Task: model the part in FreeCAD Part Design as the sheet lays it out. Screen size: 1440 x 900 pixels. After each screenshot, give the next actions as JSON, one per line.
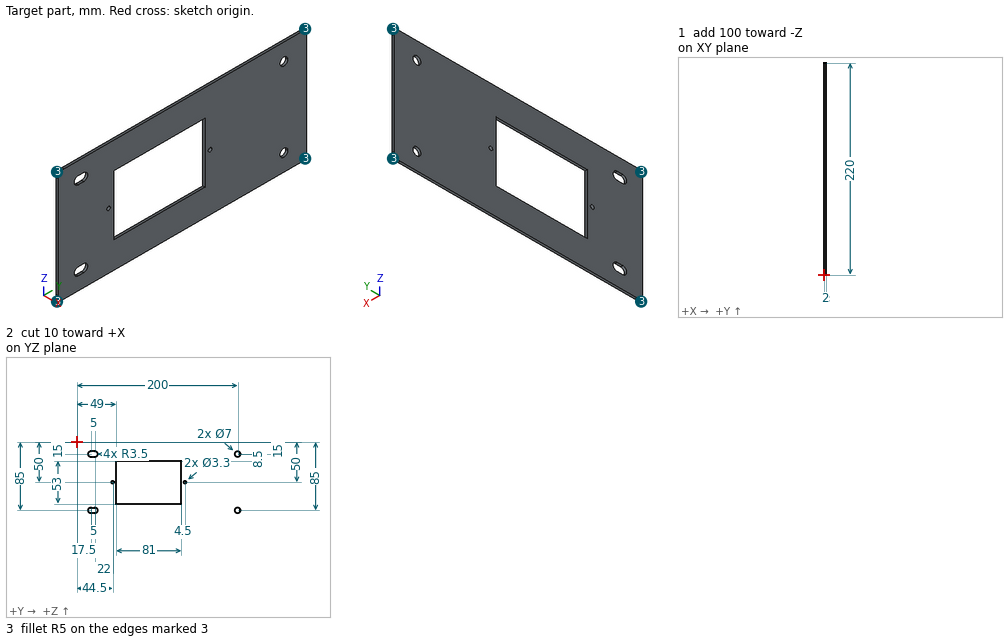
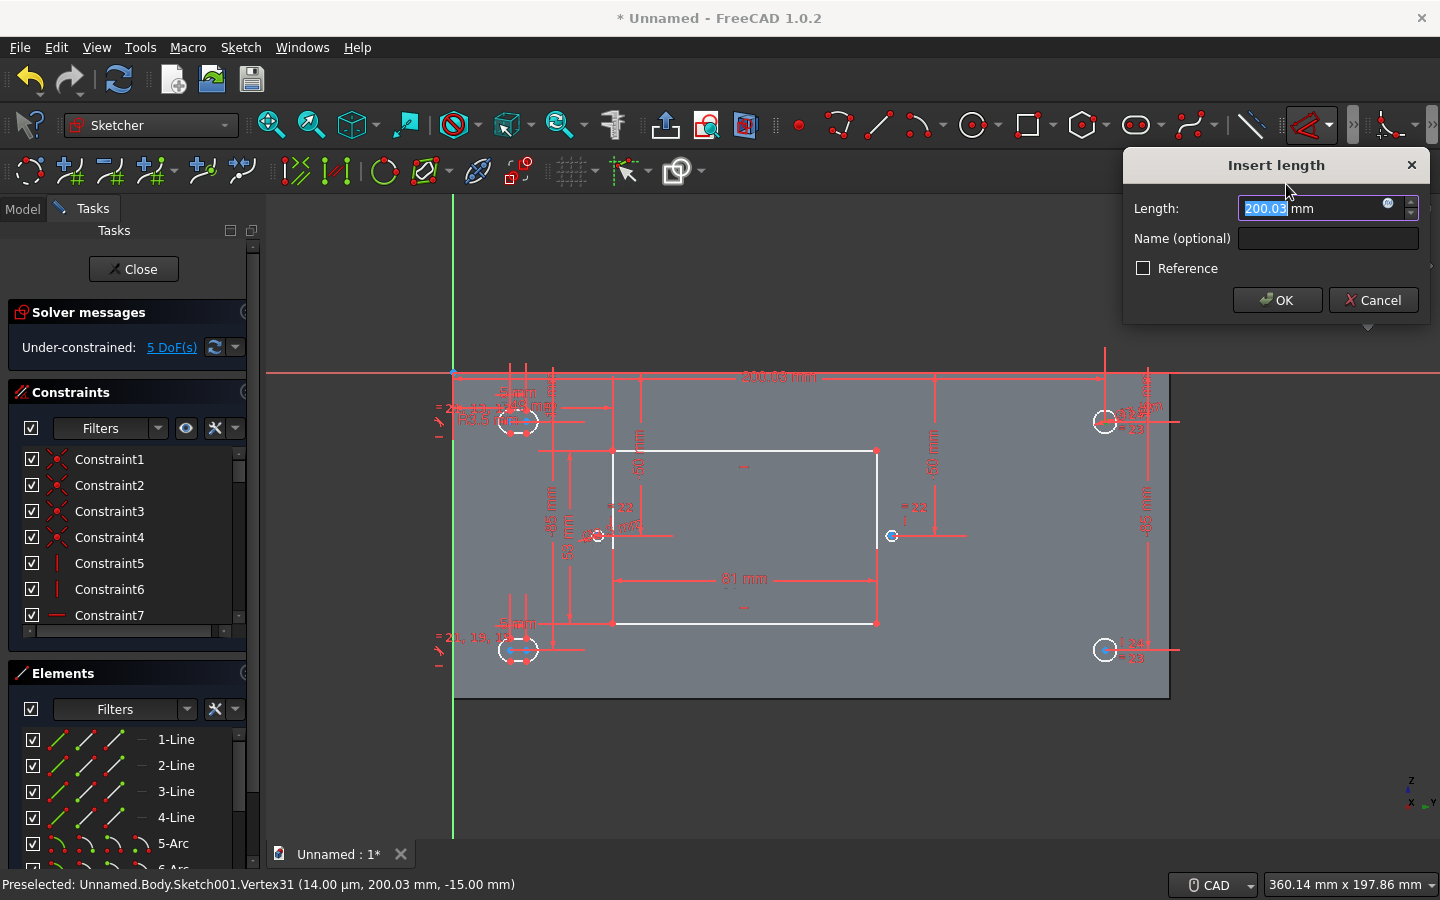
{"action": "type", "text": "200"}
{"action": "key", "text": "Return"}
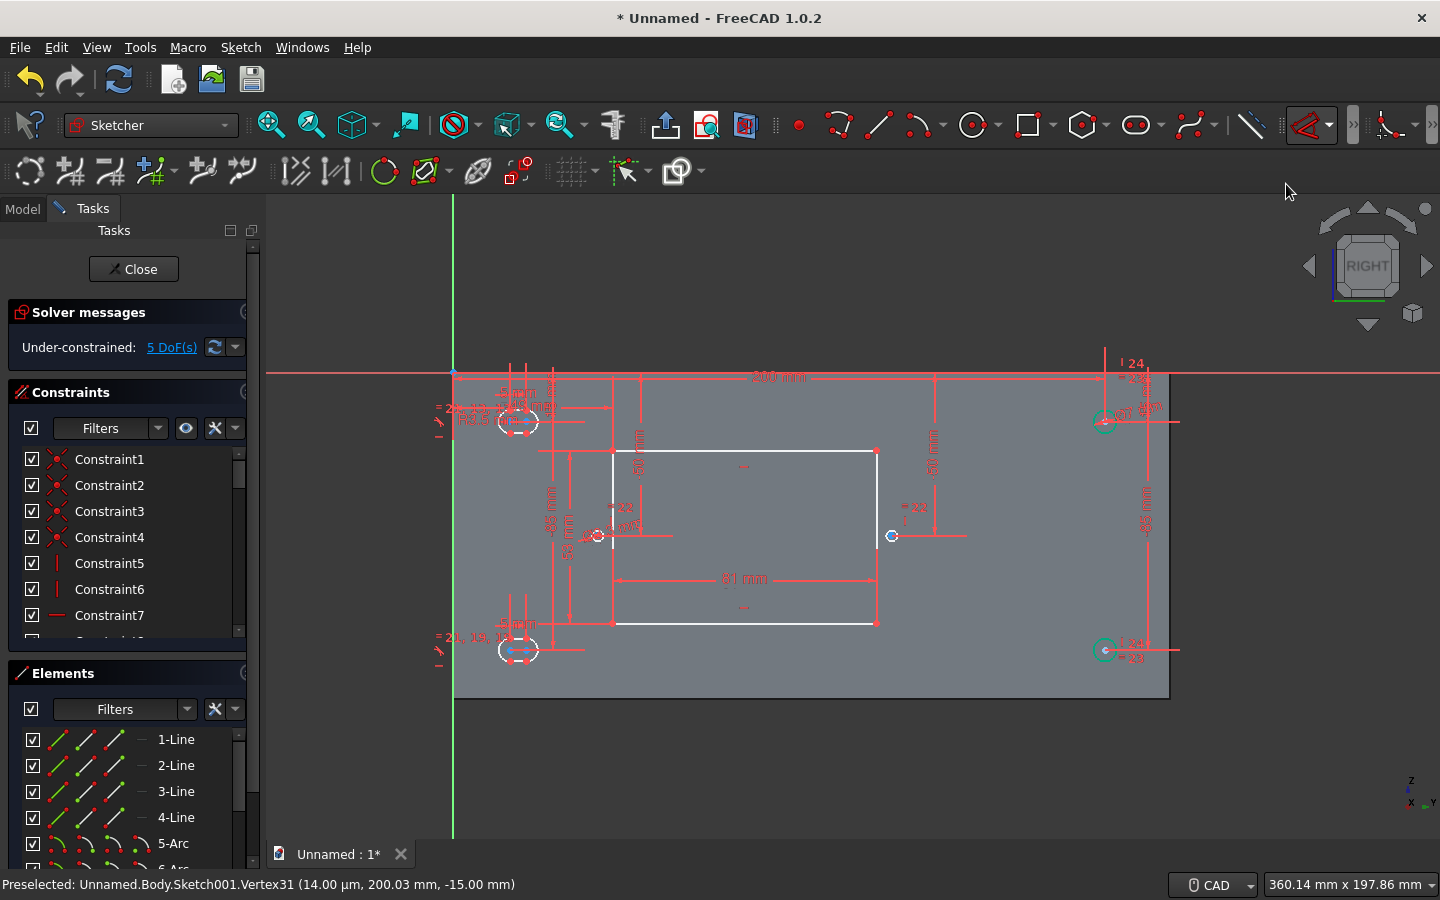
{"action": "left_click", "coordinate": [526, 433]}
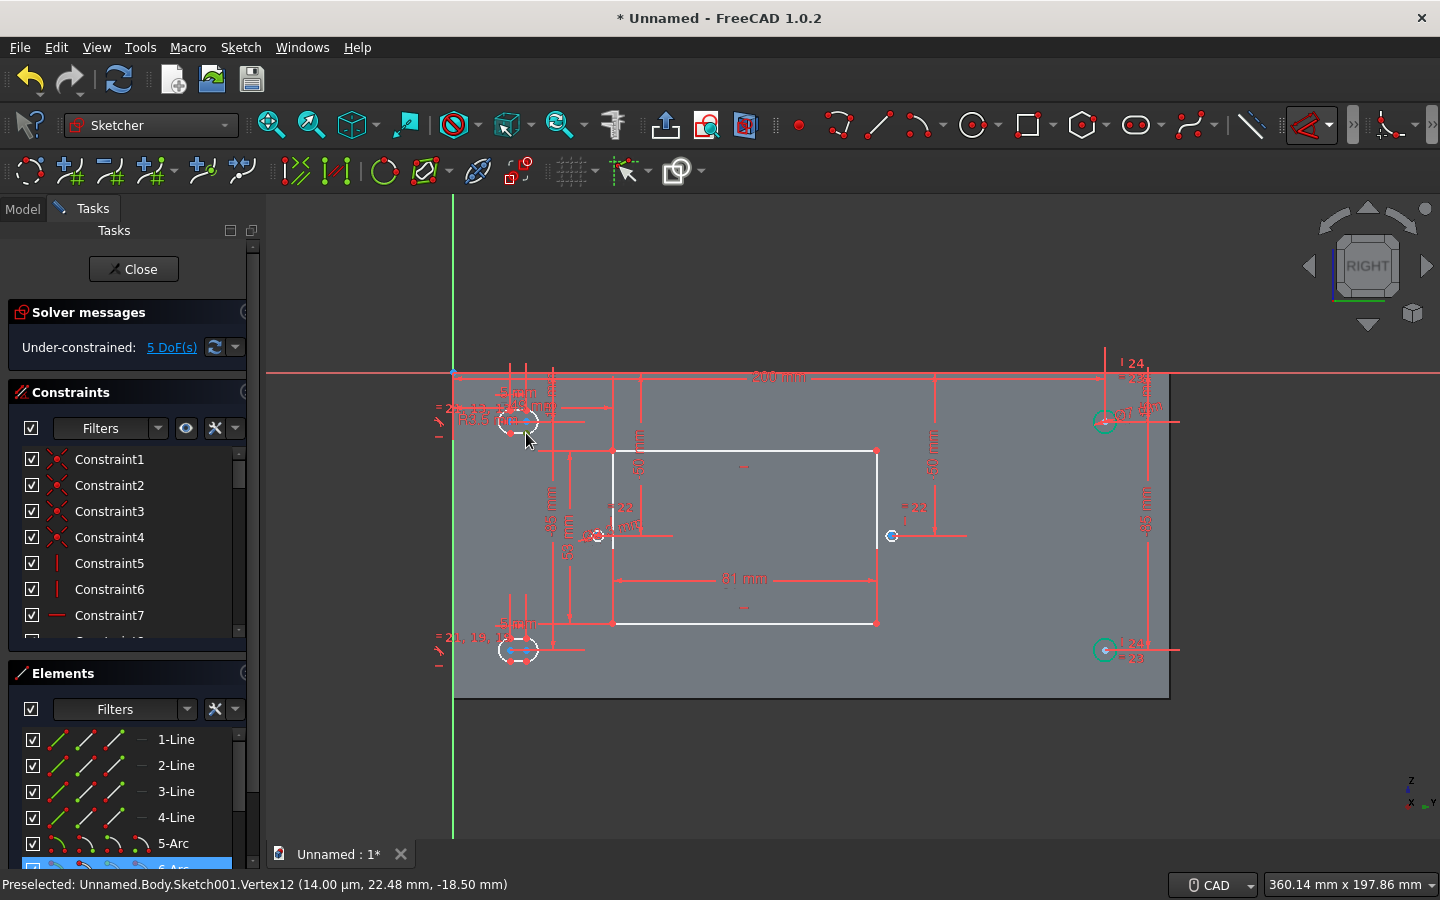
{"action": "left_click", "coordinate": [598, 536]}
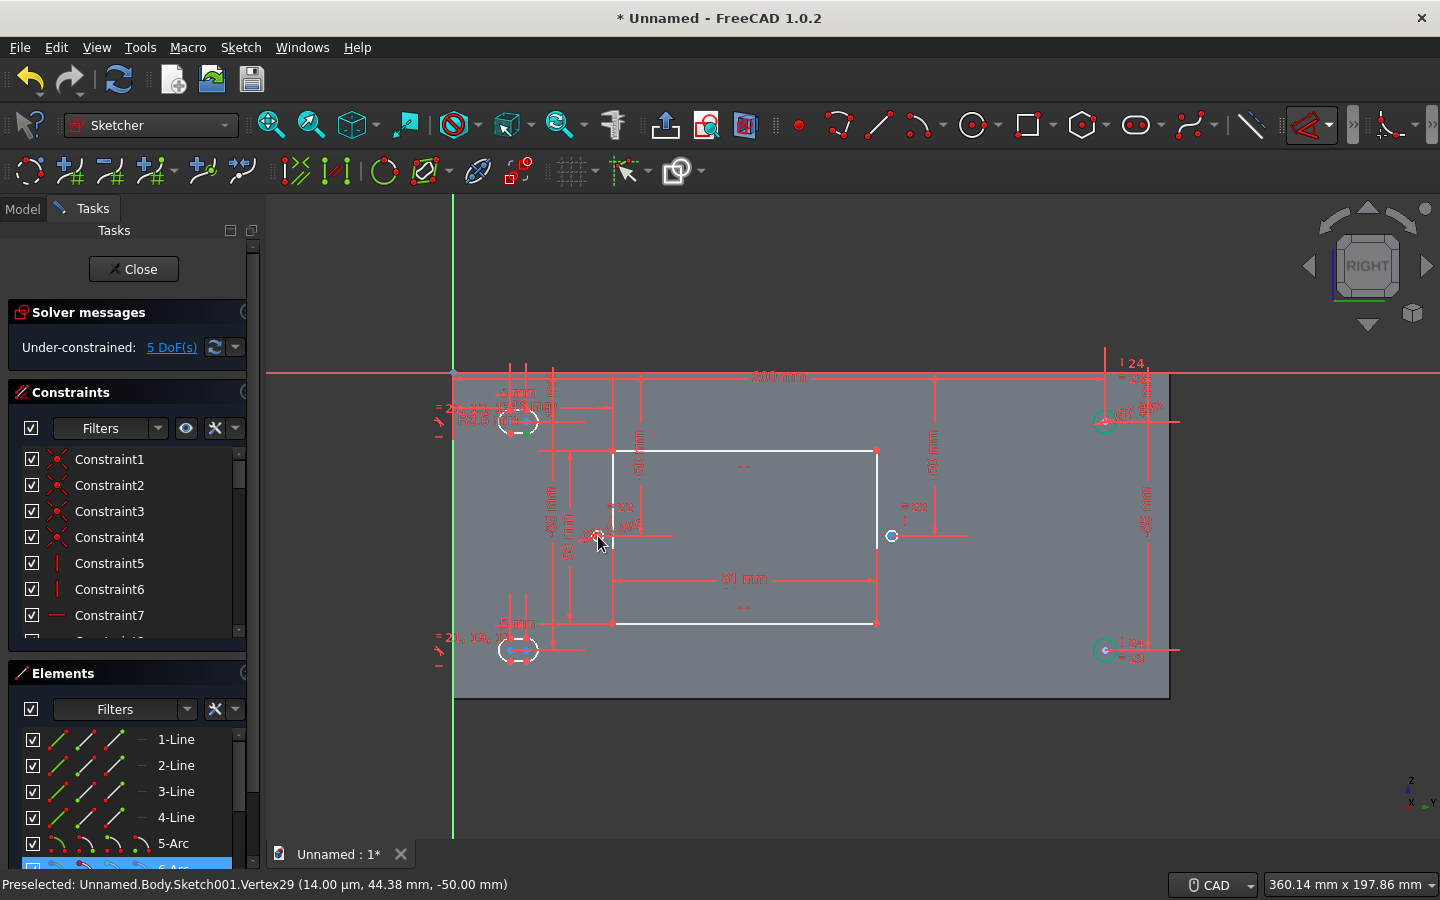
{"action": "left_click", "coordinate": [1332, 126]}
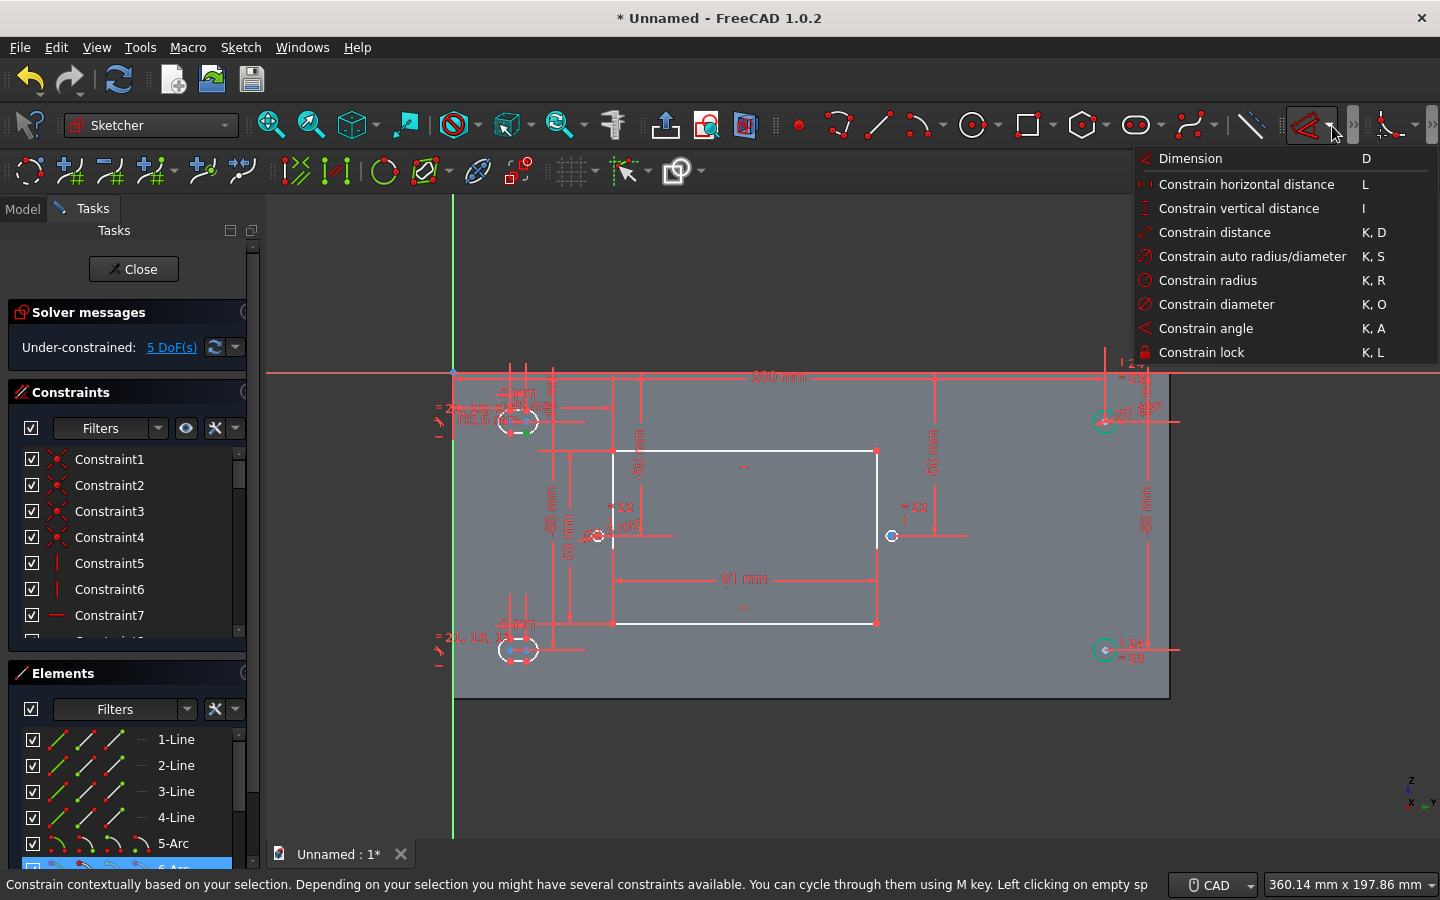
{"action": "left_click", "coordinate": [1286, 184]}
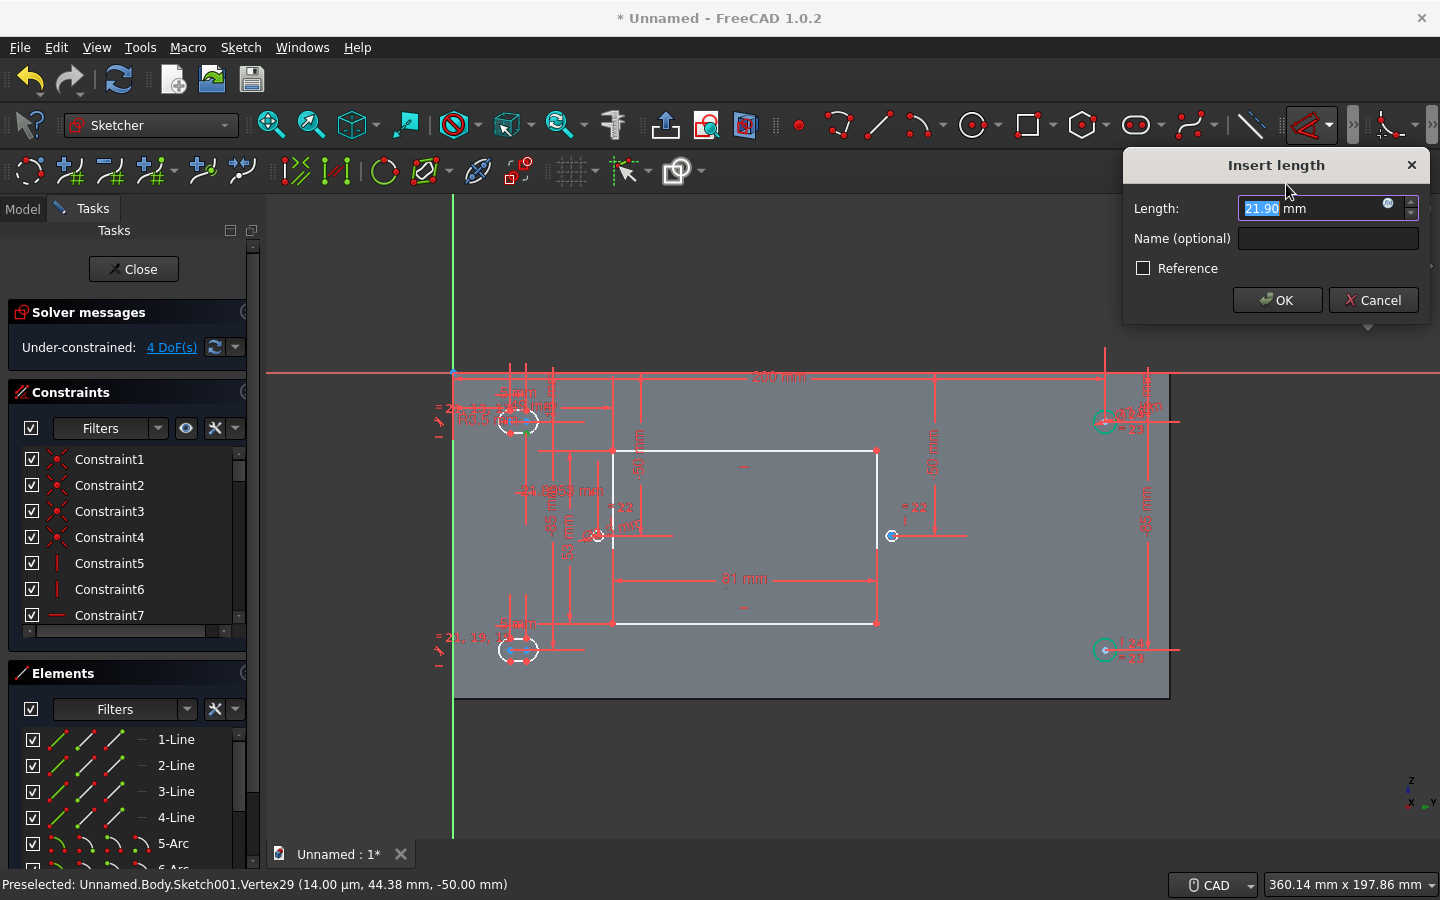
{"action": "type", "text": "22"}
{"action": "key", "text": "Return"}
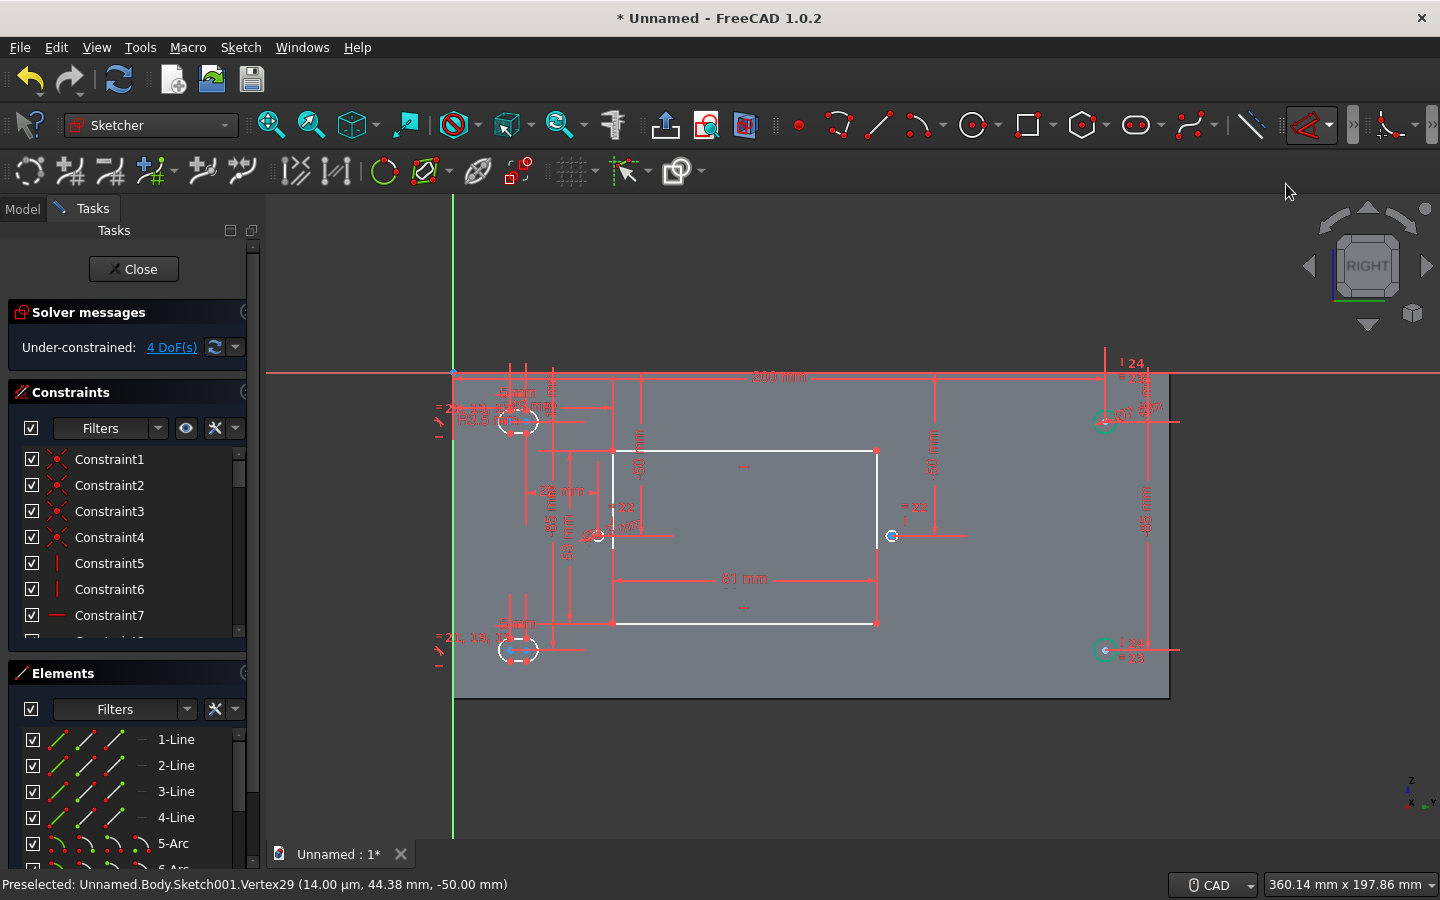
{"action": "left_click", "coordinate": [598, 536]}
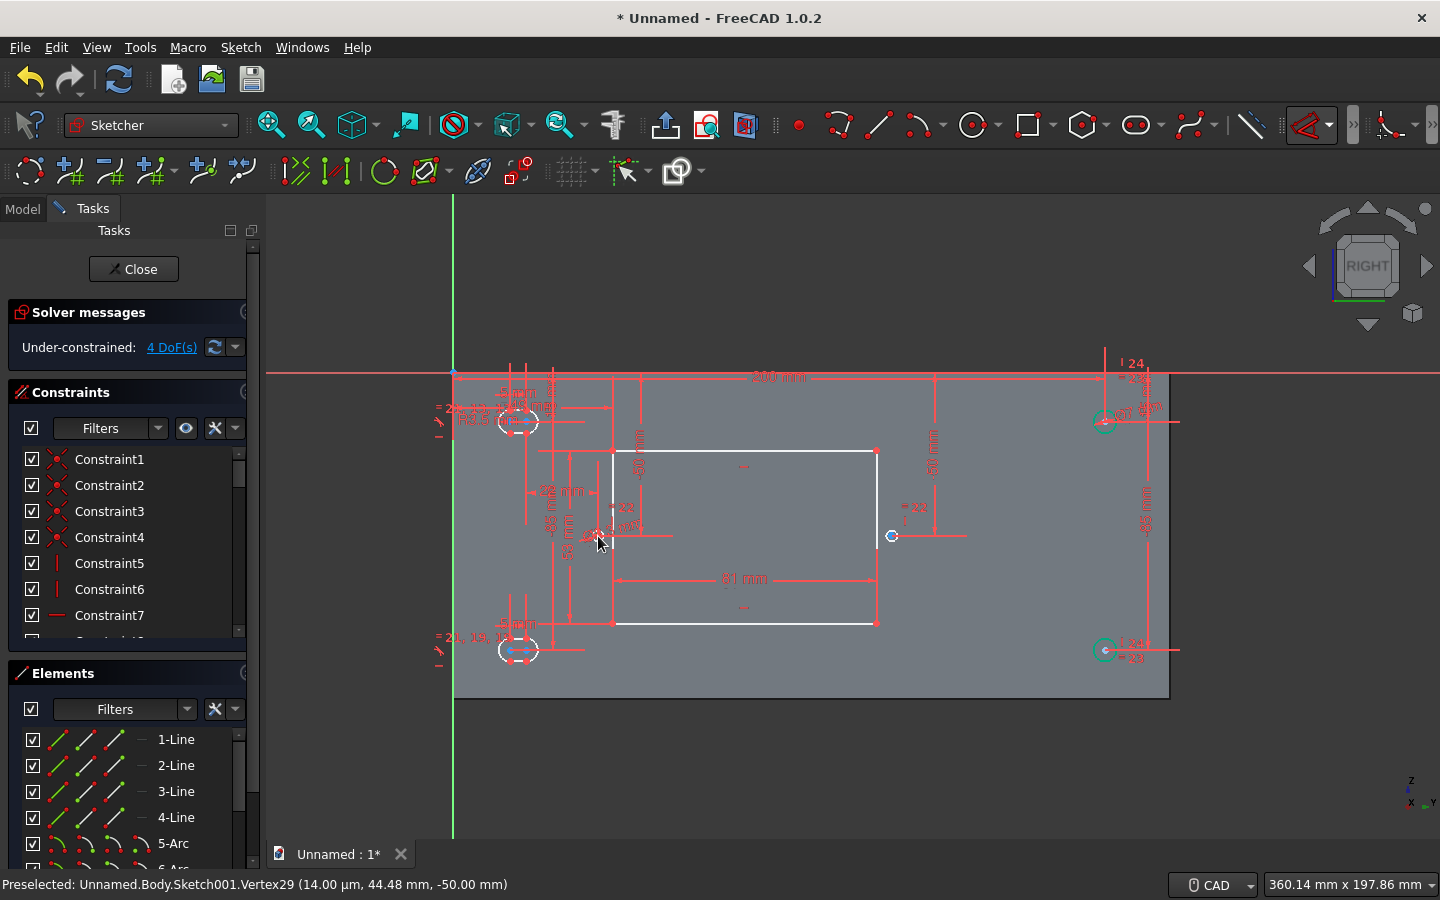
{"action": "left_click", "coordinate": [1332, 126]}